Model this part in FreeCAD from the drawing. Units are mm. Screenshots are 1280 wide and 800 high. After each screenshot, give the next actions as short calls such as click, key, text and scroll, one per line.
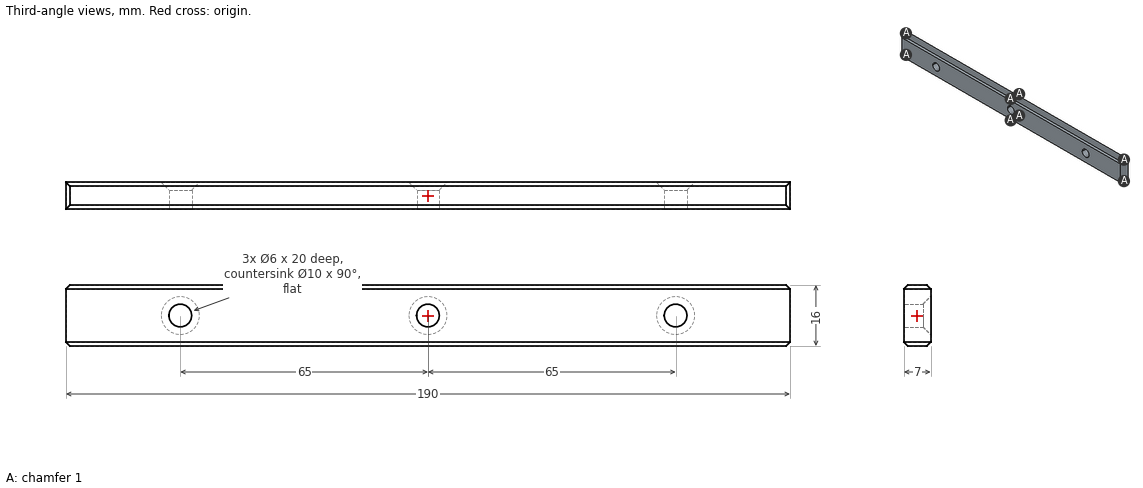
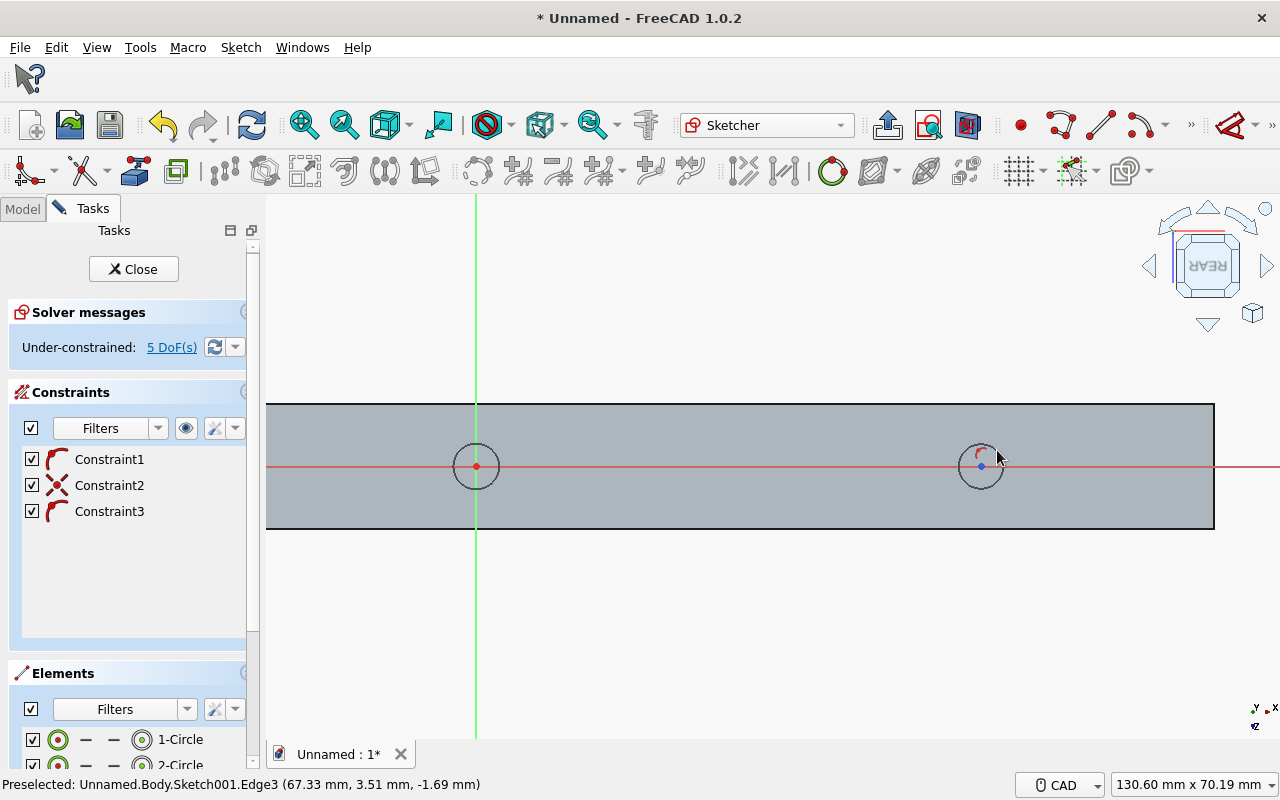
scroll(982, 467, down, 3)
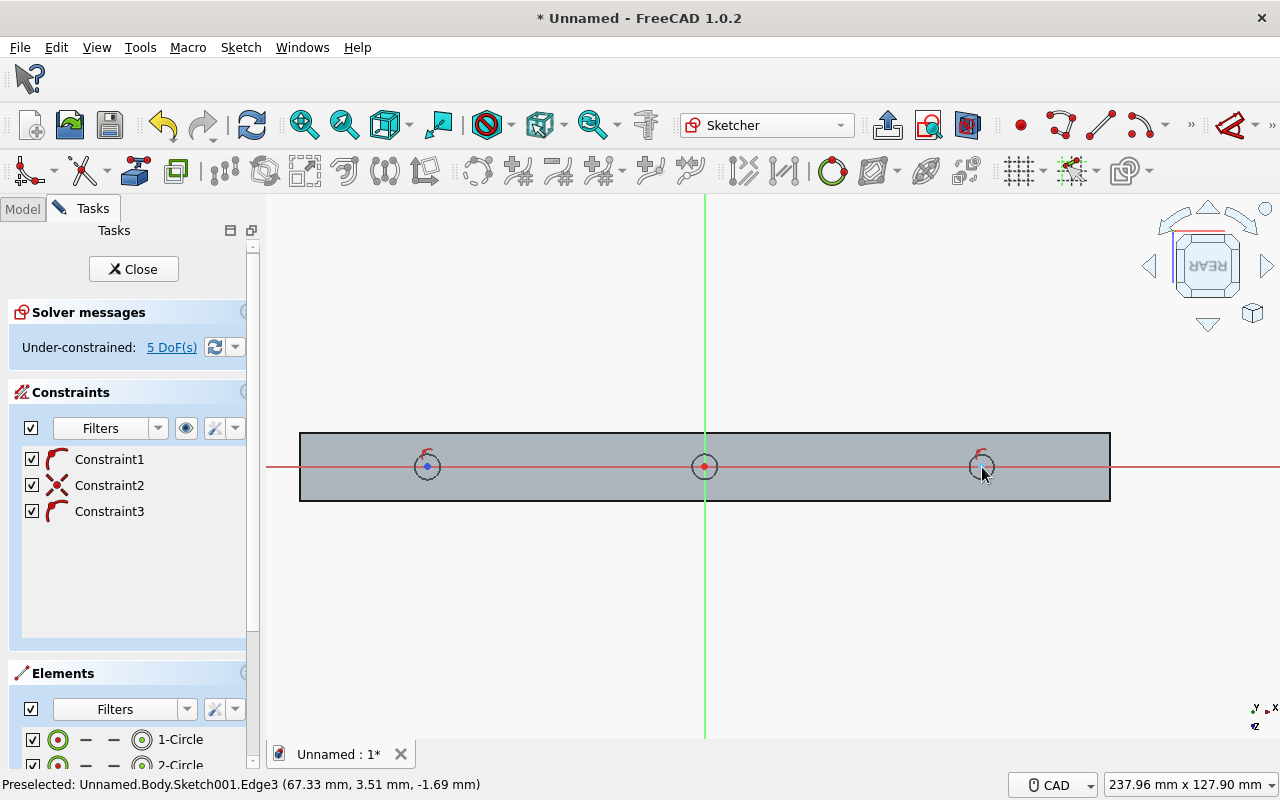
scroll(436, 458, up, 3)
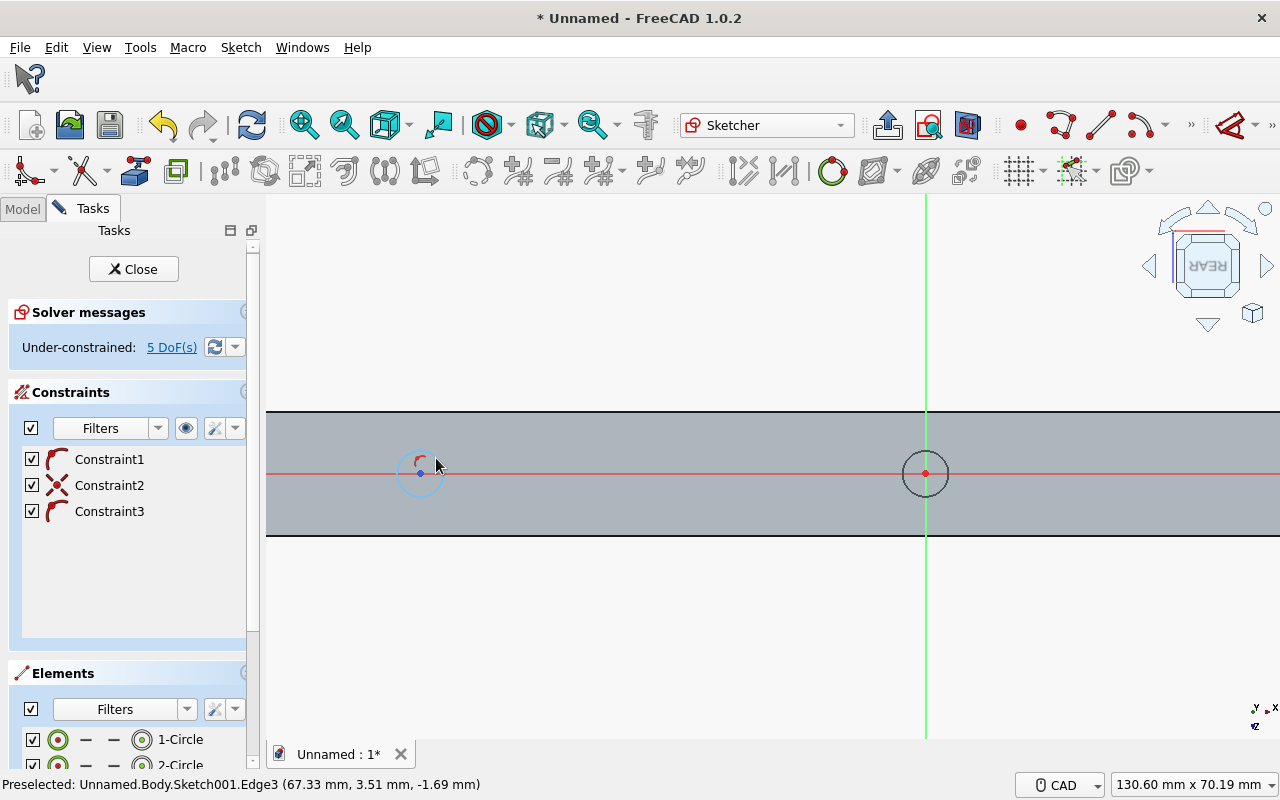
click(437, 458)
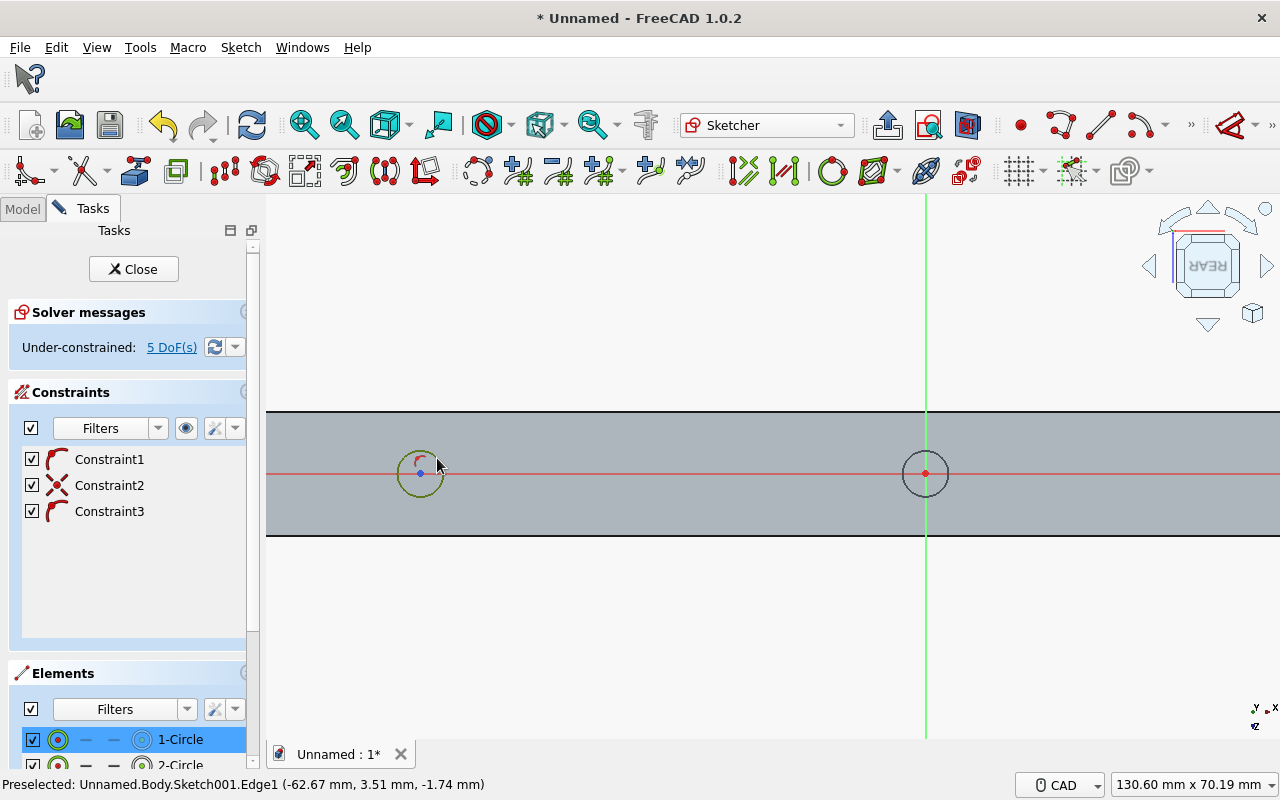
click(942, 458)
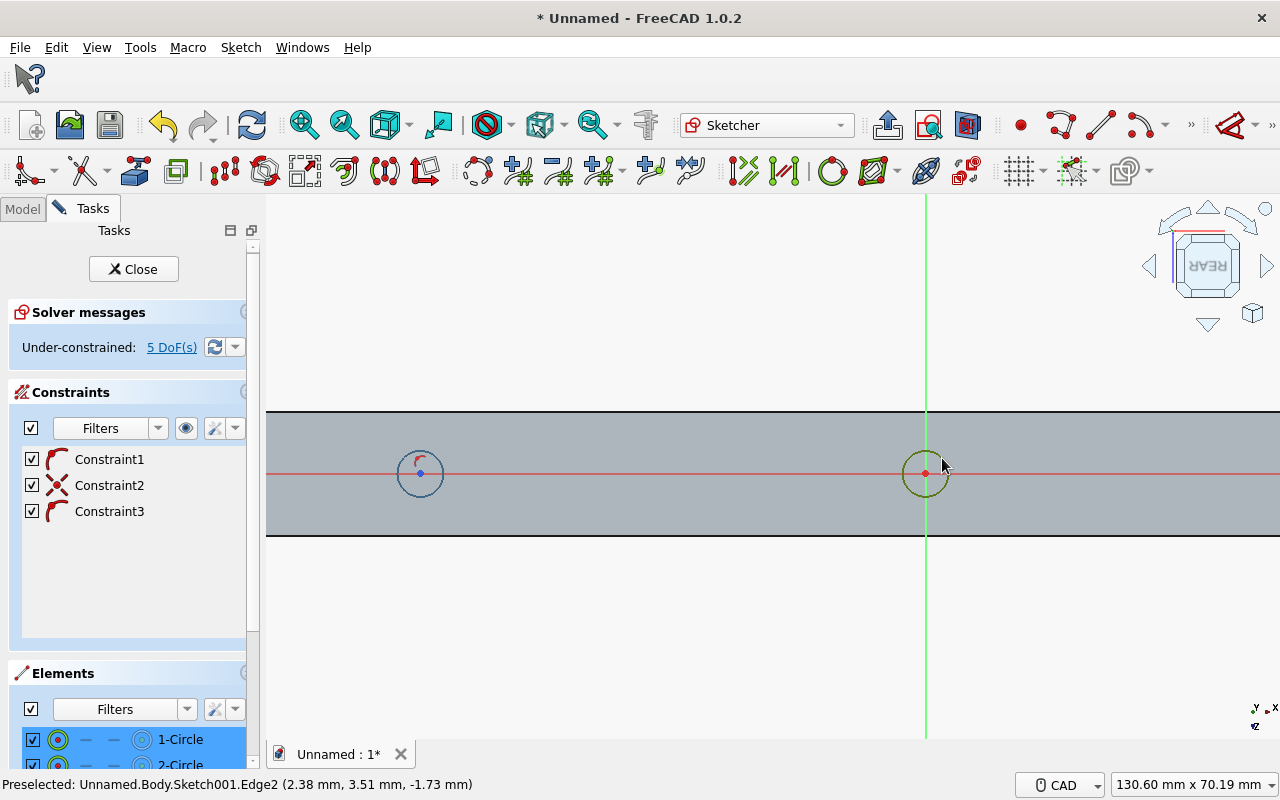
scroll(436, 457, down, 3)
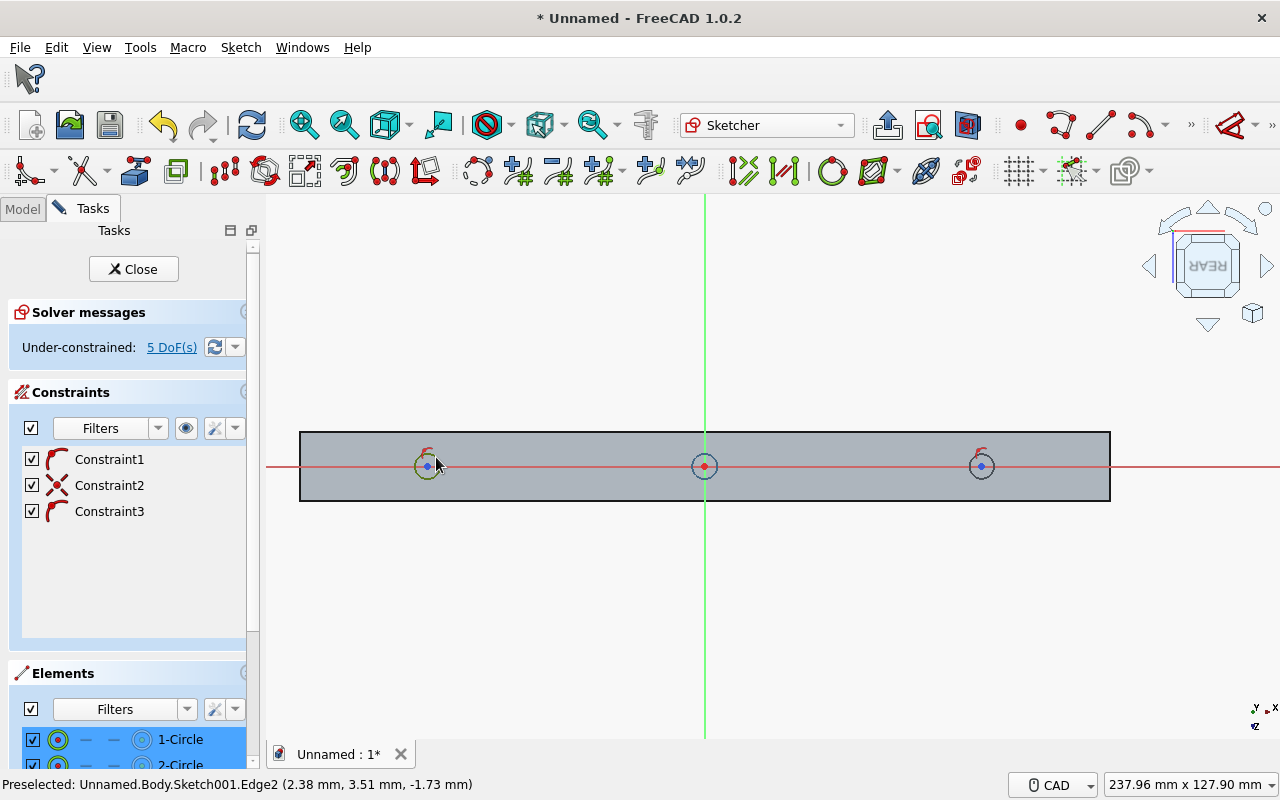
scroll(990, 458, up, 3)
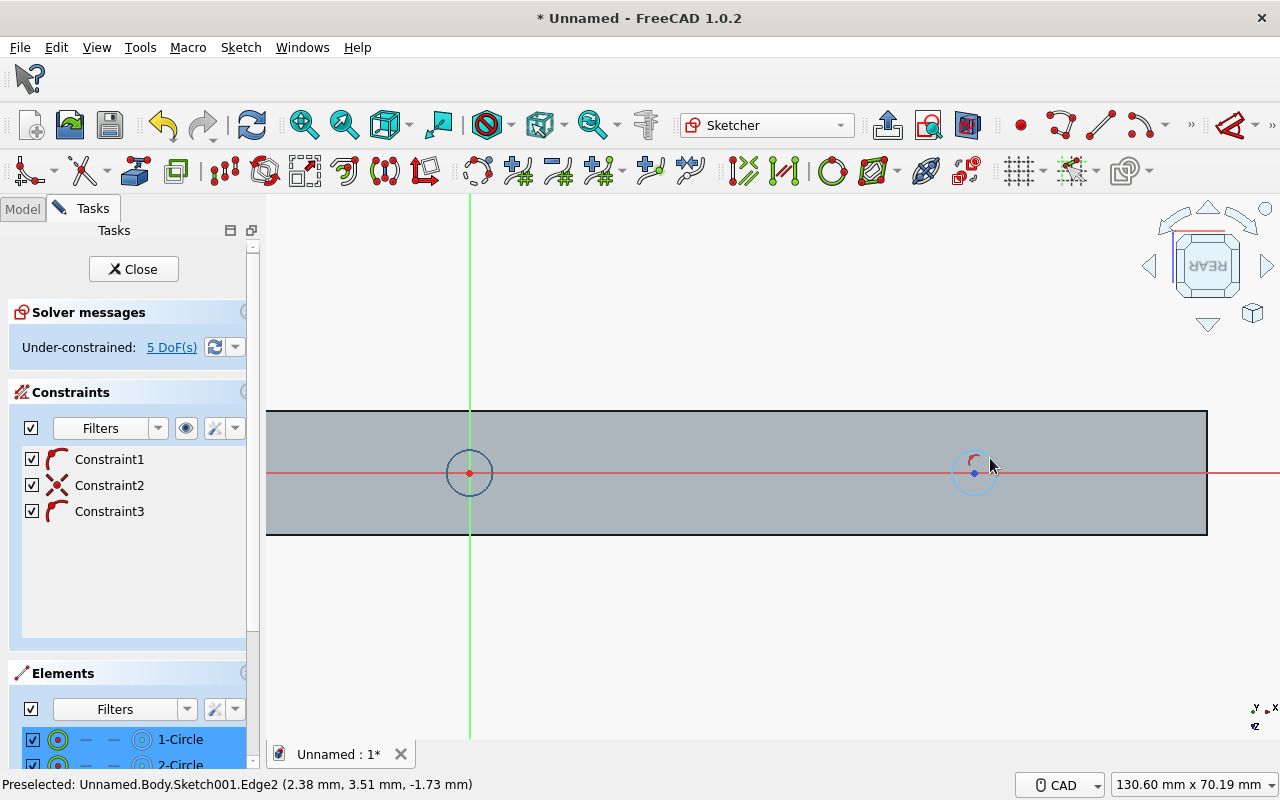
click(990, 457)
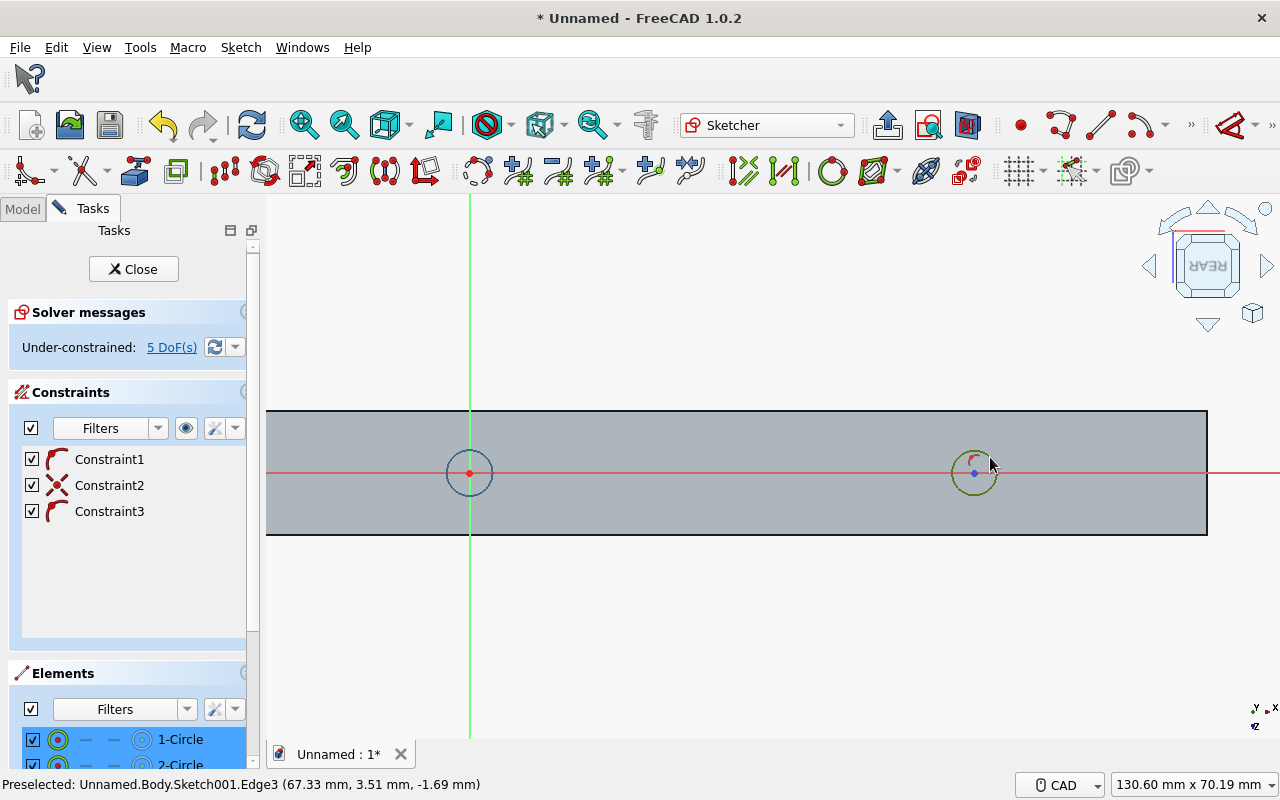
key(e)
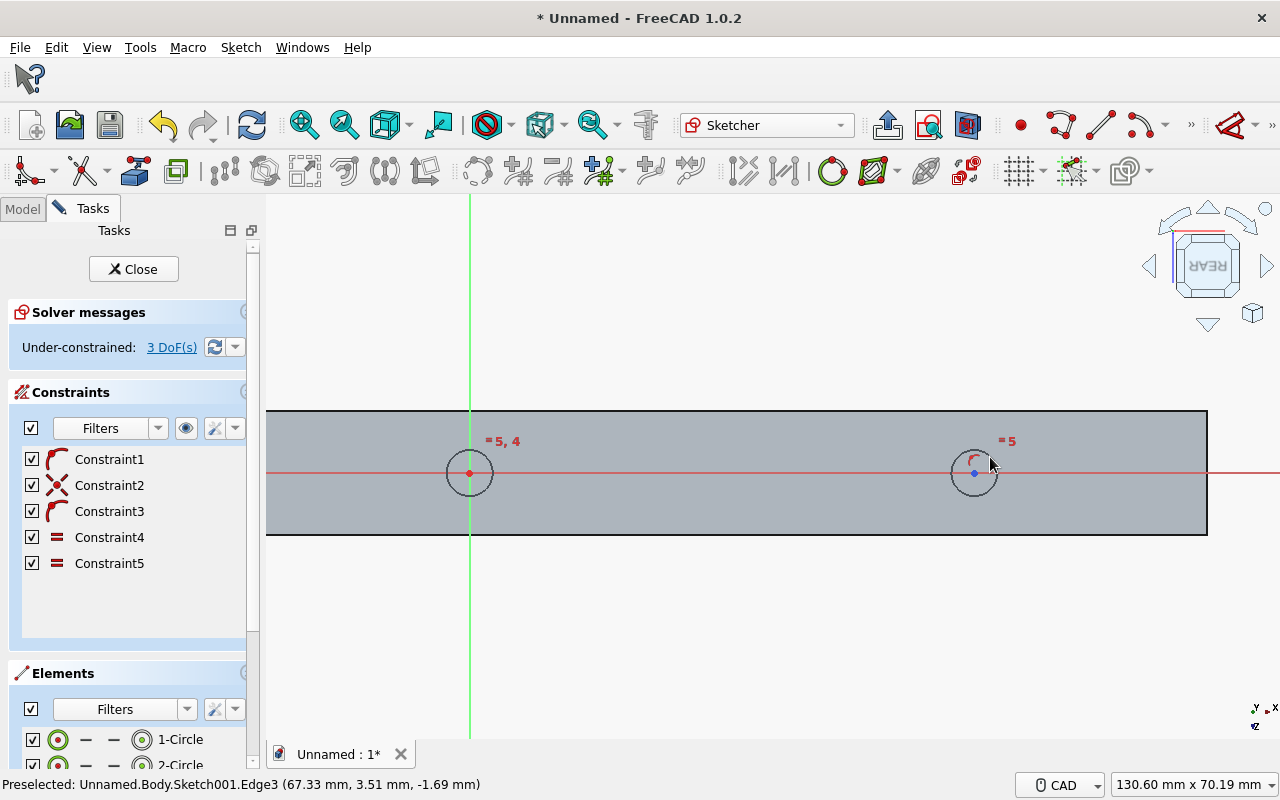
click(1230, 126)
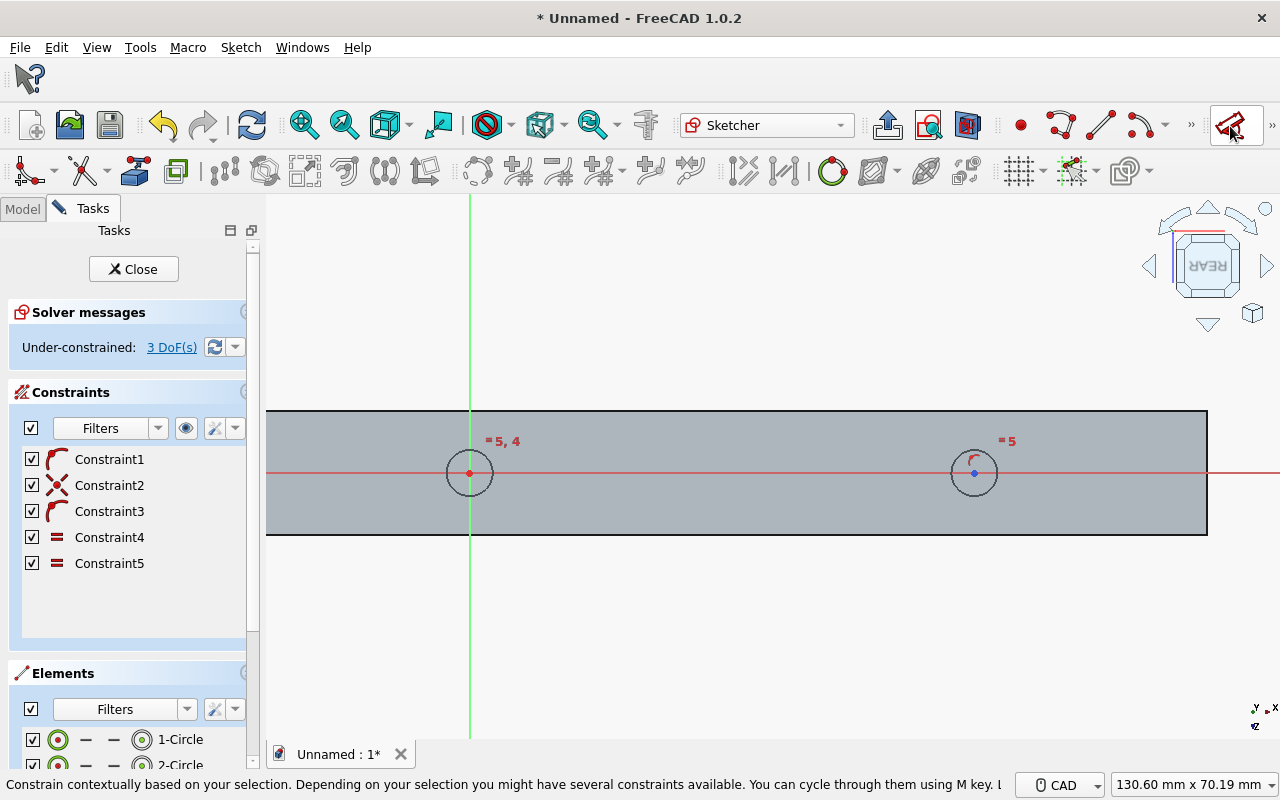
scroll(990, 458, down, 3)